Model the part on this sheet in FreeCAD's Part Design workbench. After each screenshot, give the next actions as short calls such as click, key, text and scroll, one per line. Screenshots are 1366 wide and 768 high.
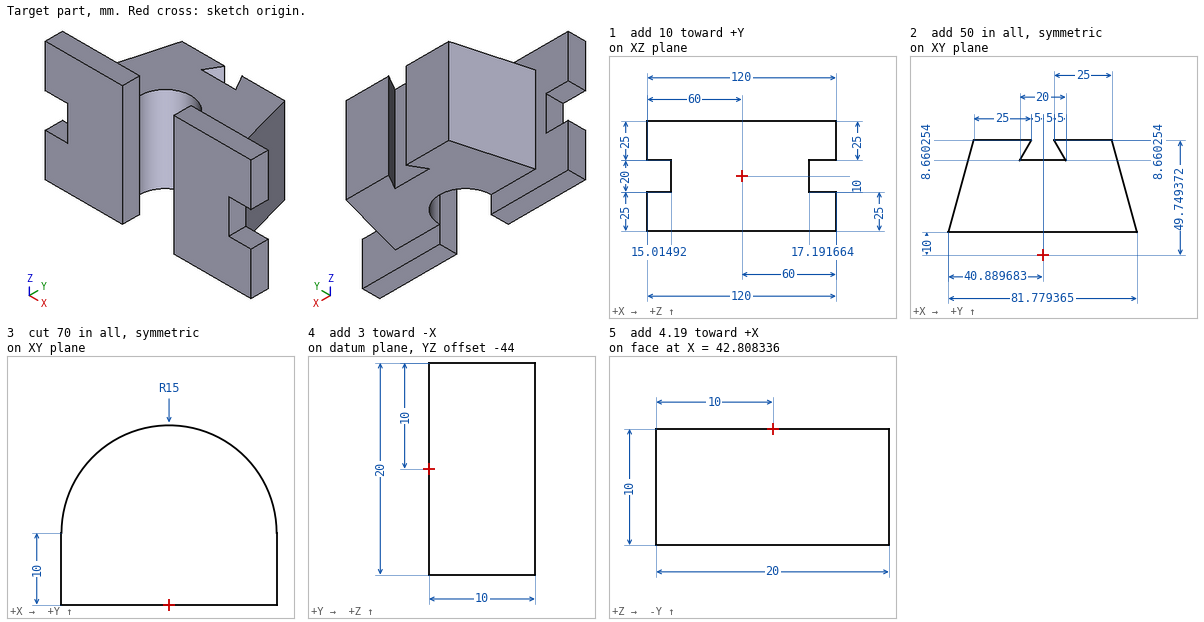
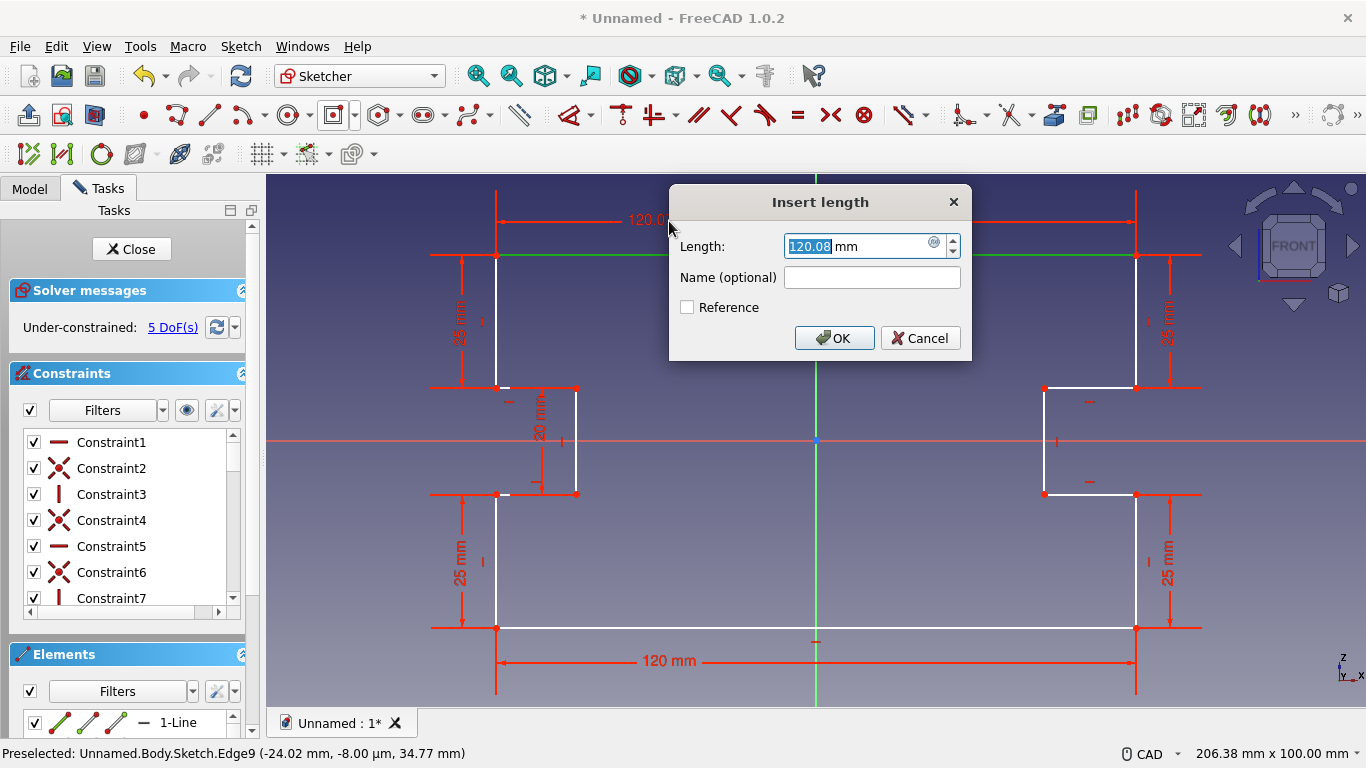
text(120)
key(Return)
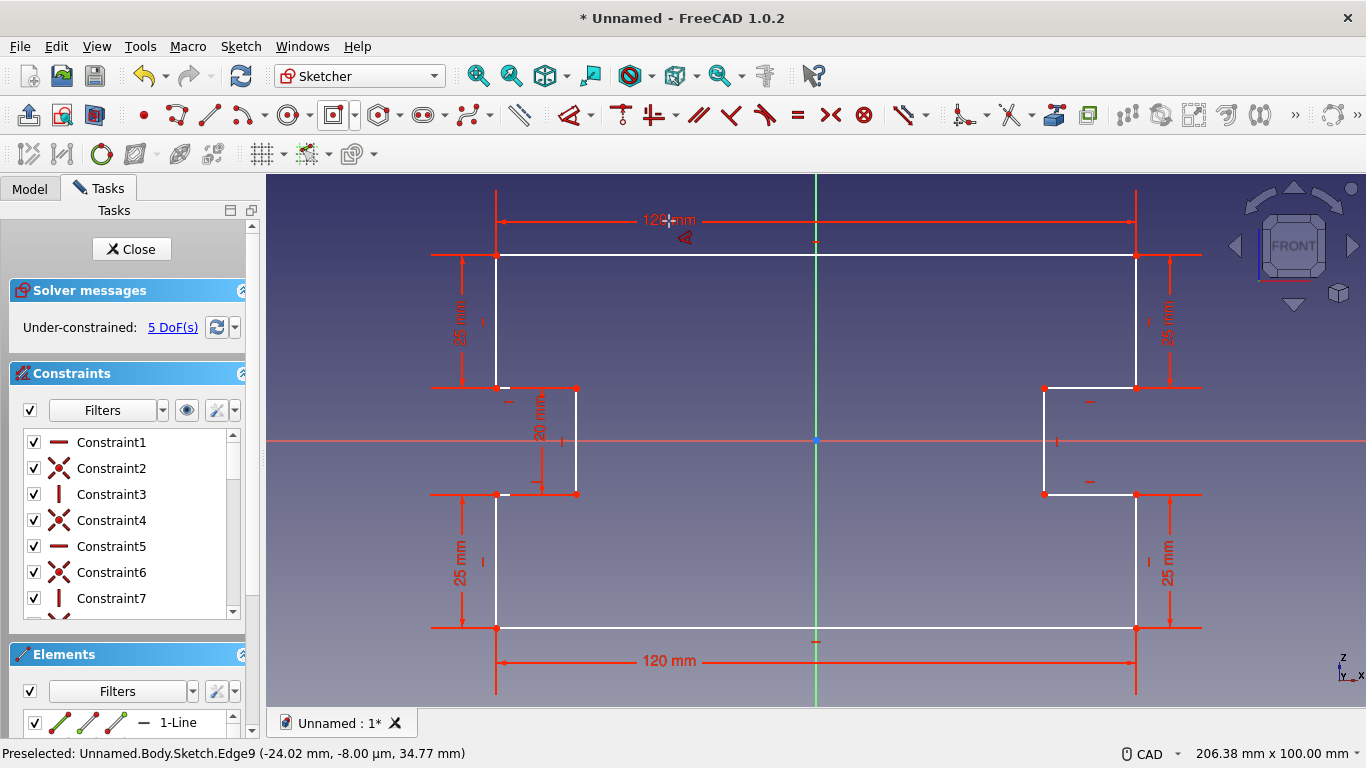
click(1044, 495)
click(1078, 468)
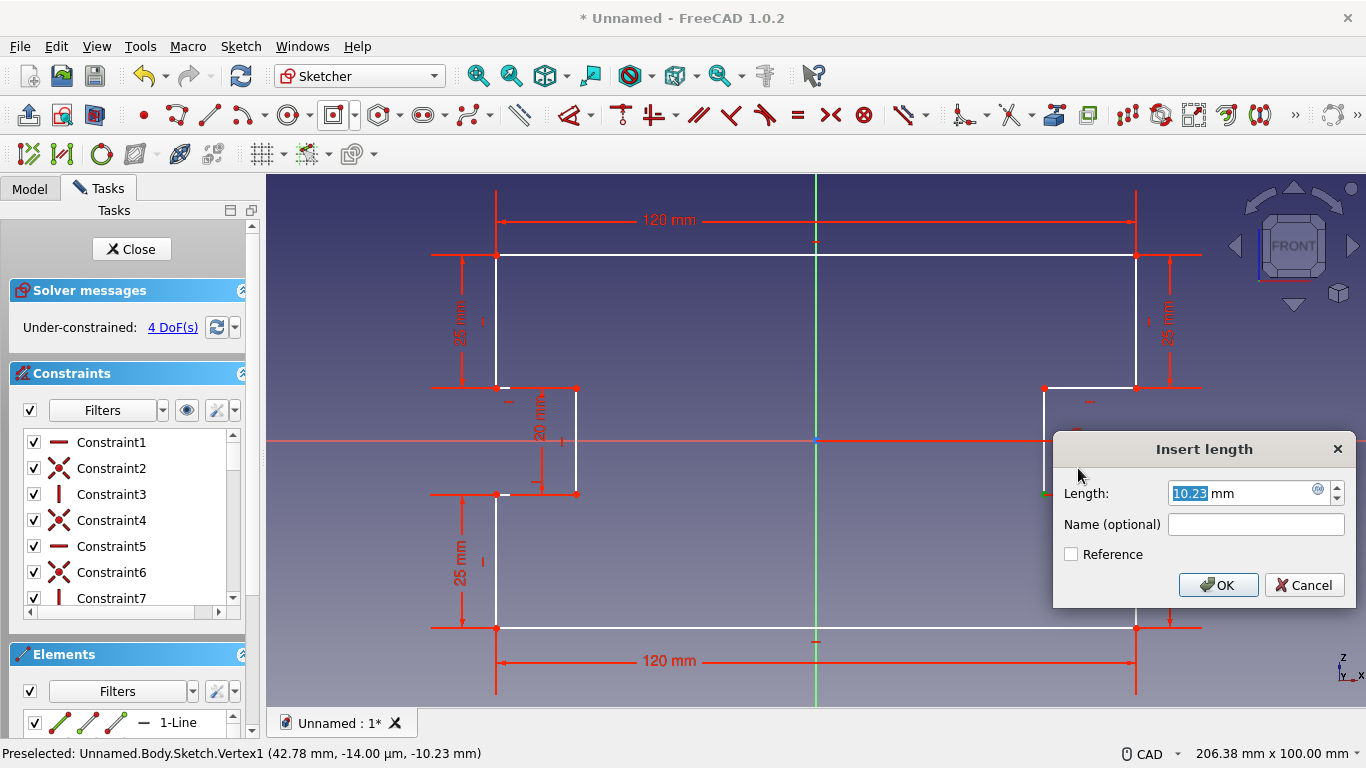
text(10)
key(Return)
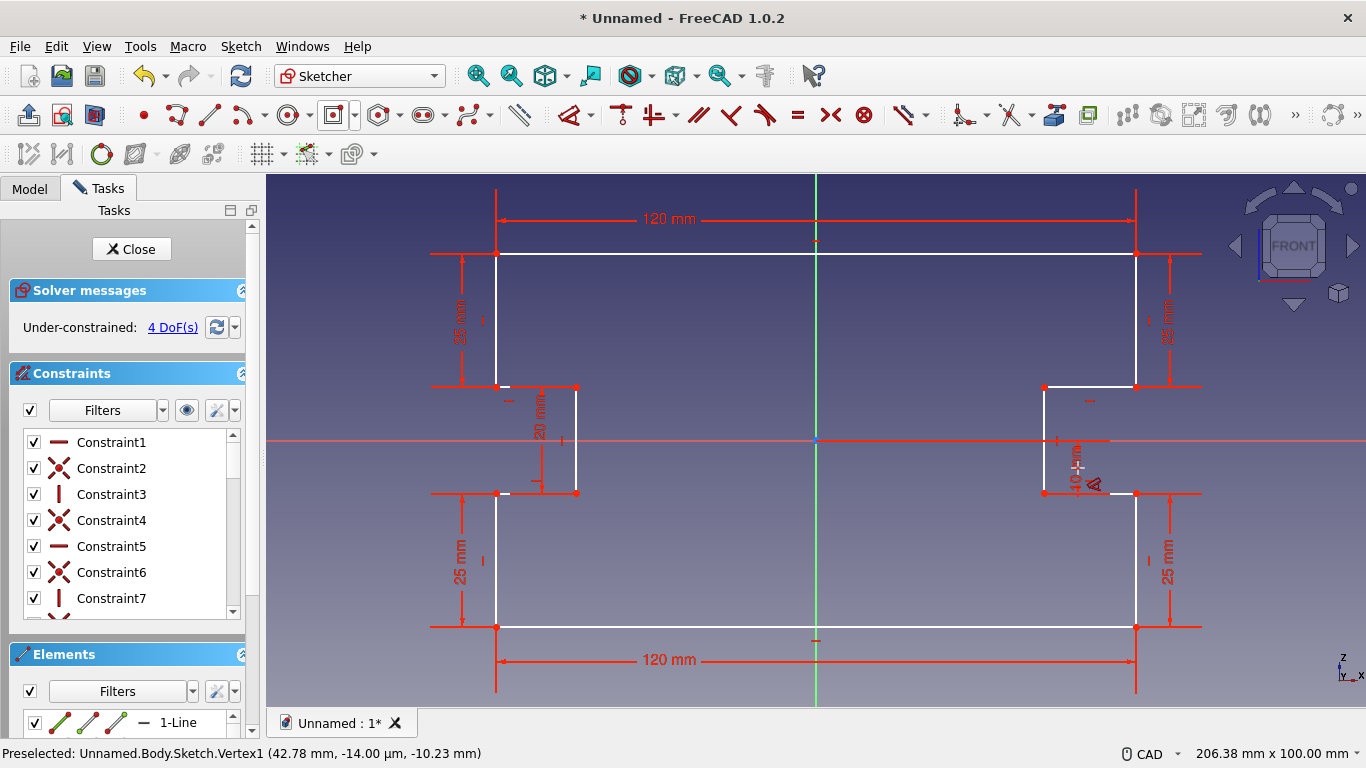
click(1136, 494)
click(976, 528)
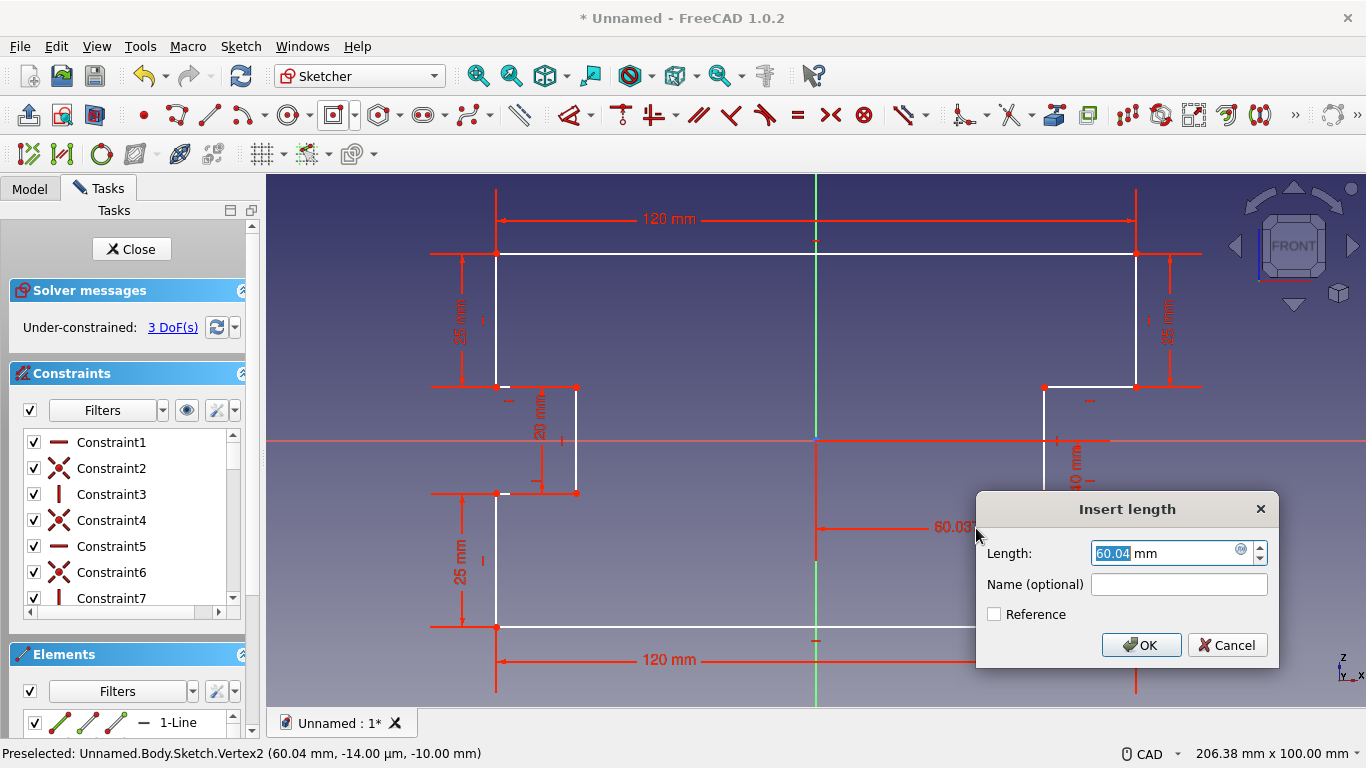
text(60)
key(Return)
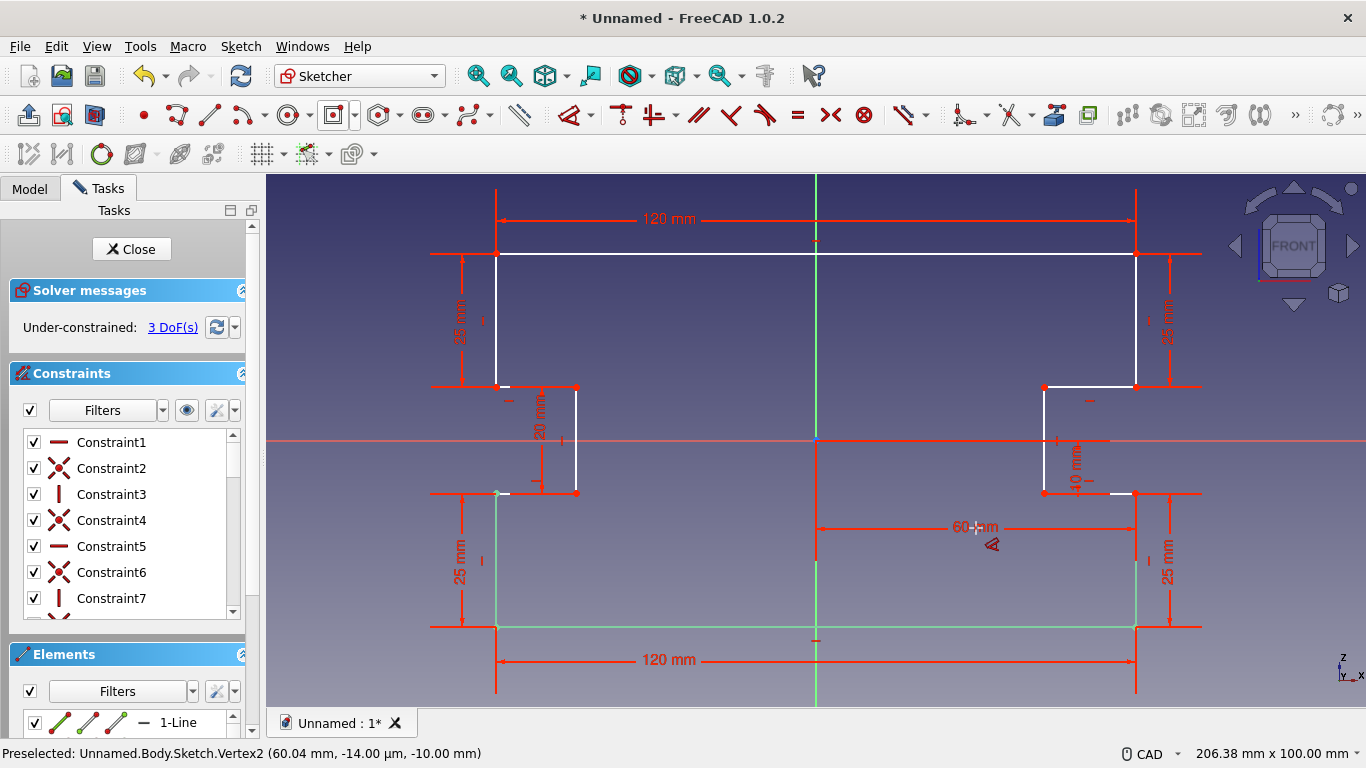
click(496, 387)
click(656, 353)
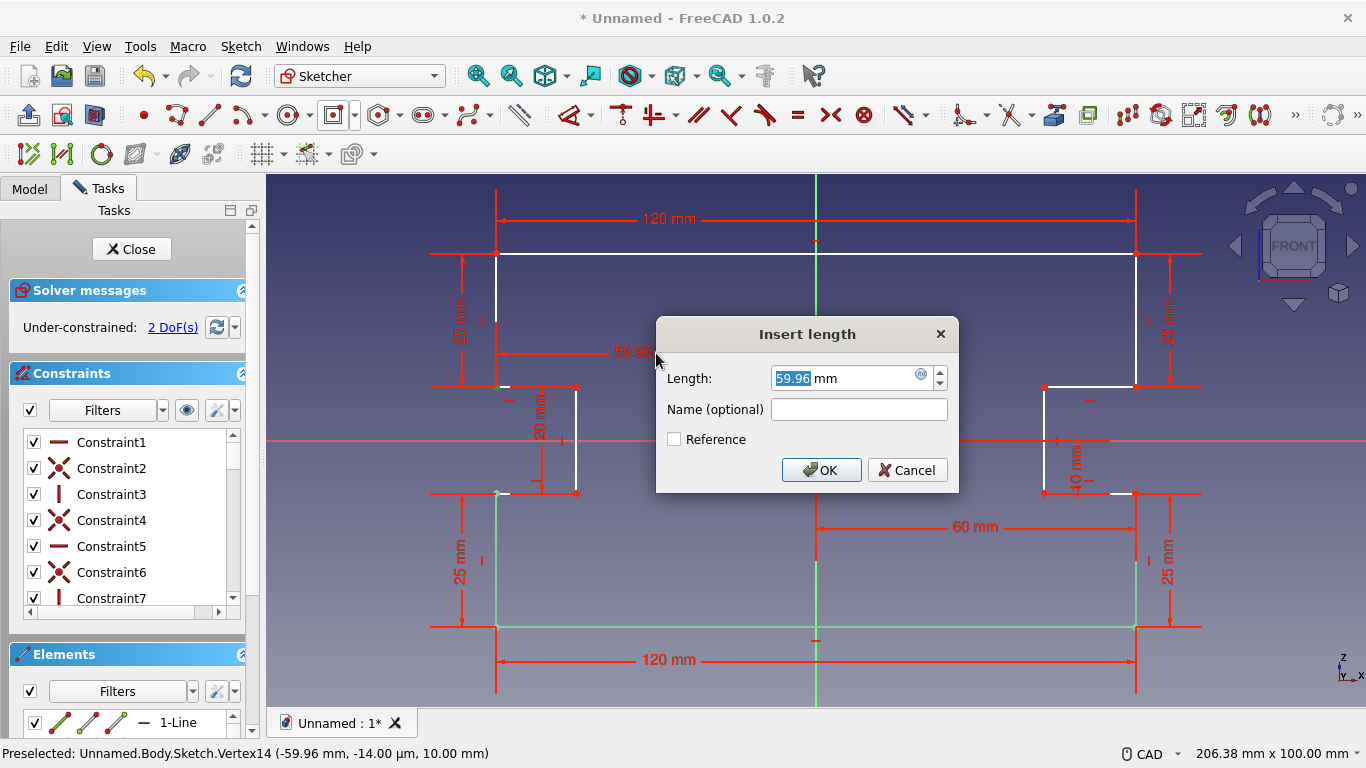
text(60)
key(Return)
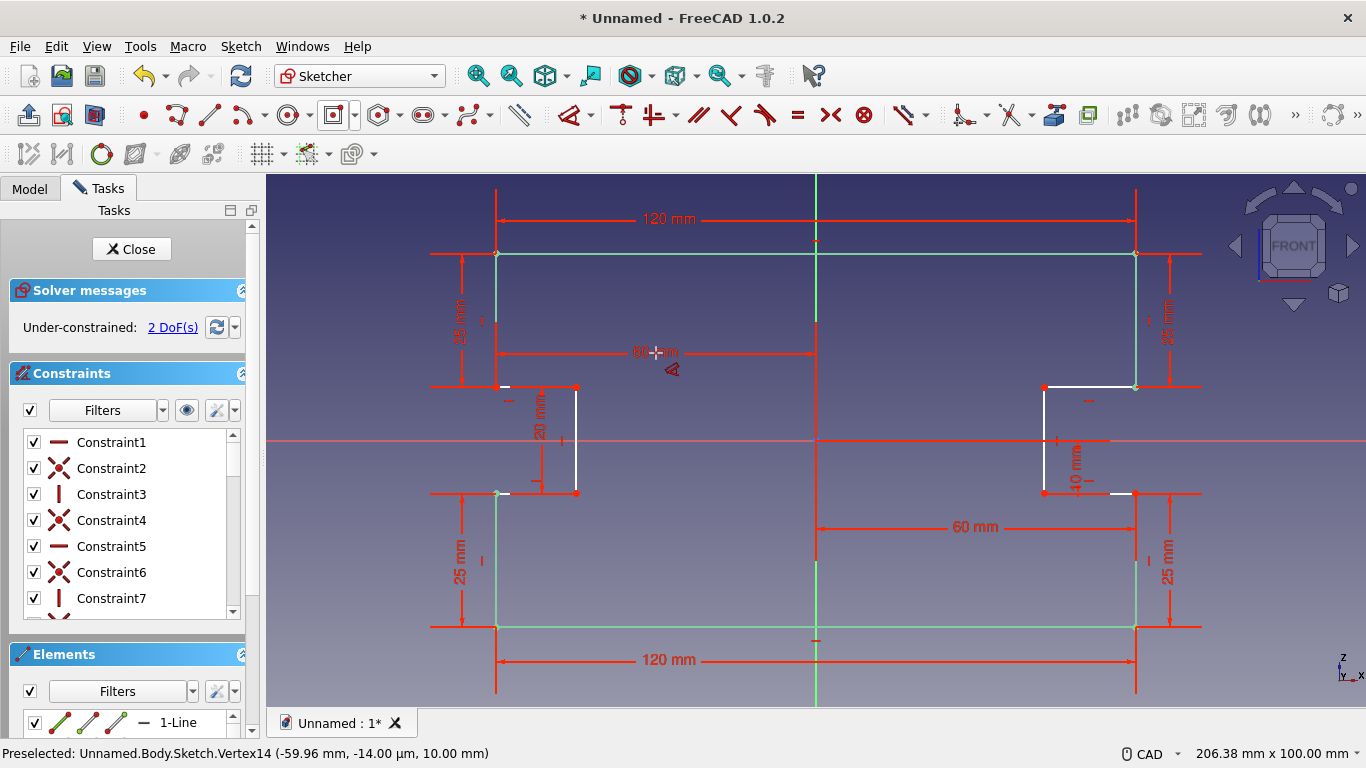
click(520, 494)
click(536, 528)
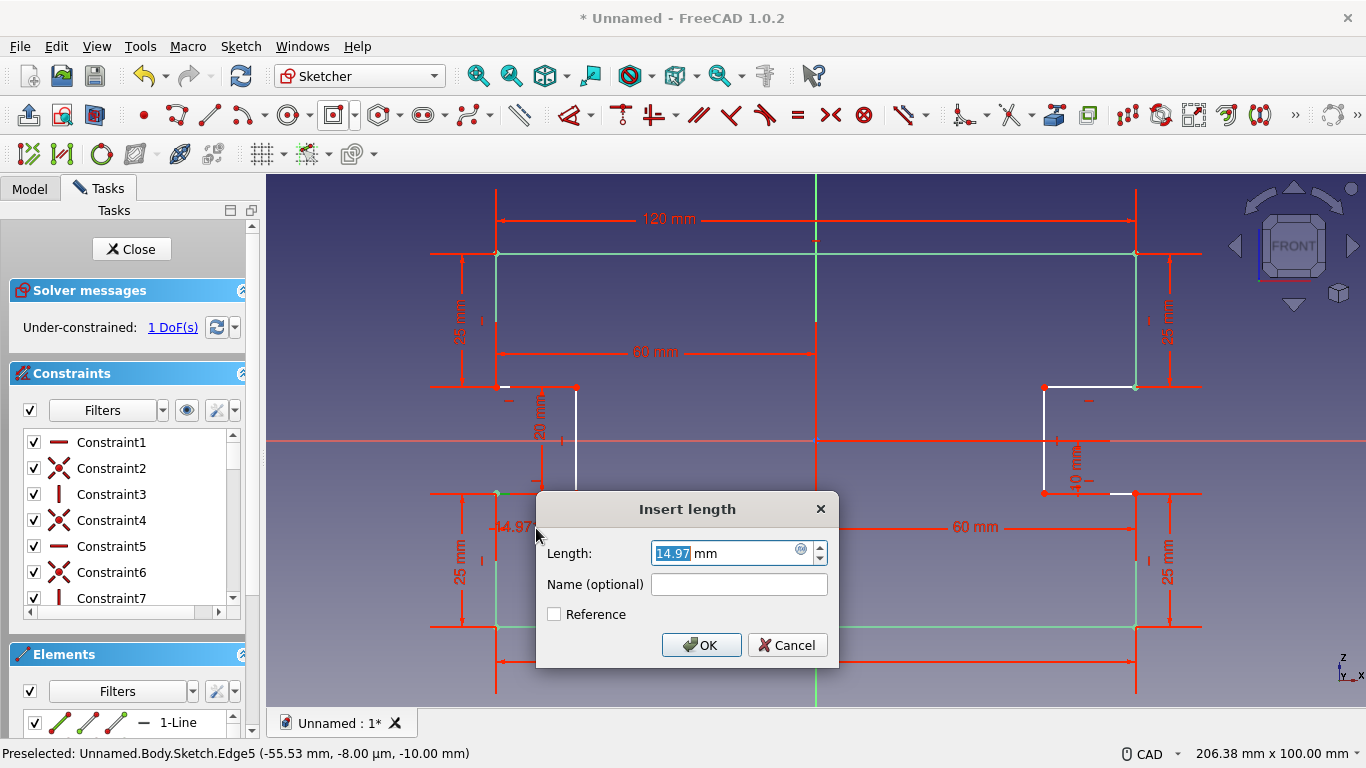
text(15.01492)
key(Return)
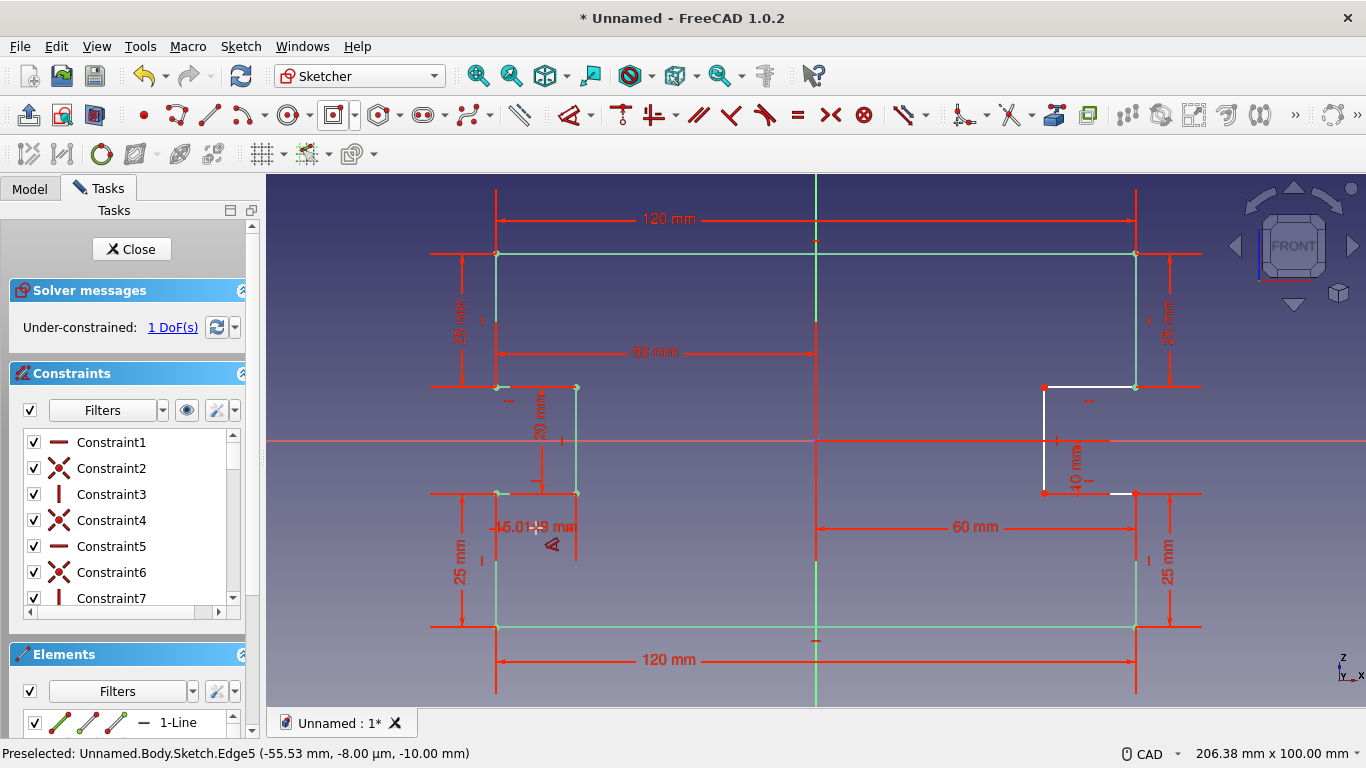
click(1072, 494)
click(1090, 528)